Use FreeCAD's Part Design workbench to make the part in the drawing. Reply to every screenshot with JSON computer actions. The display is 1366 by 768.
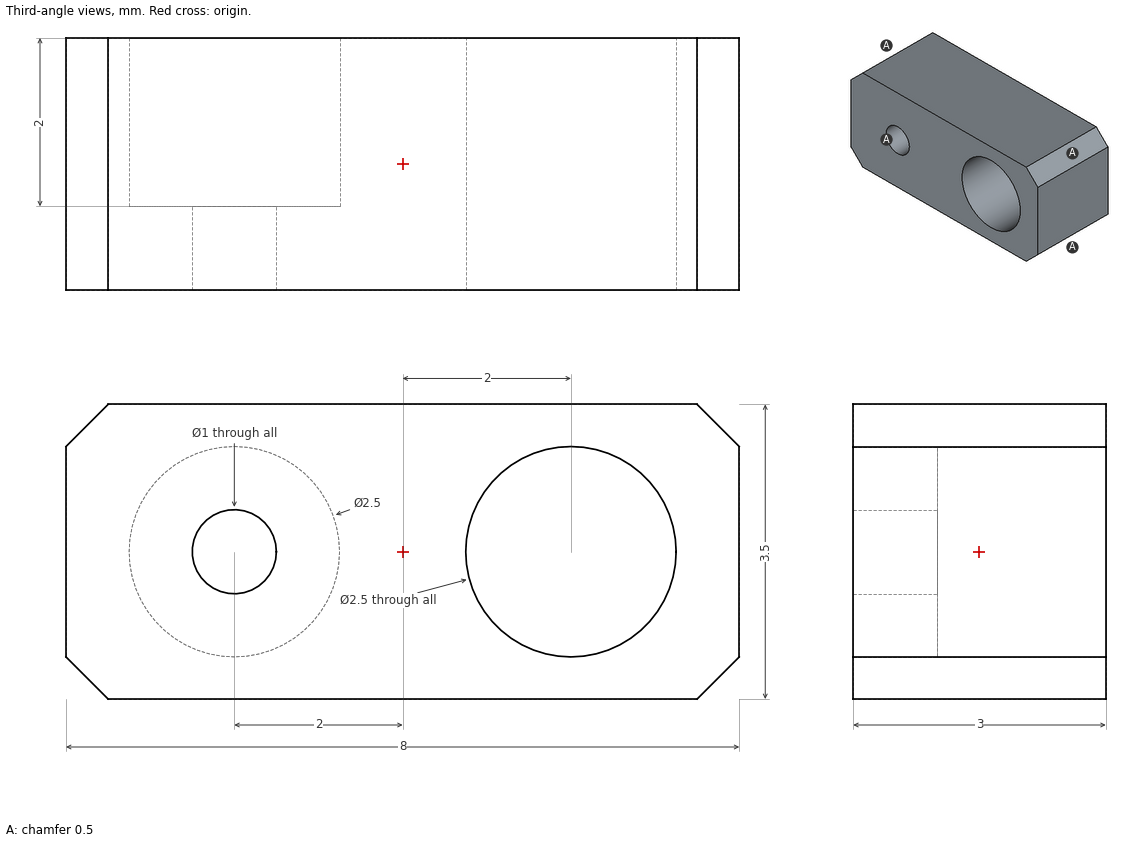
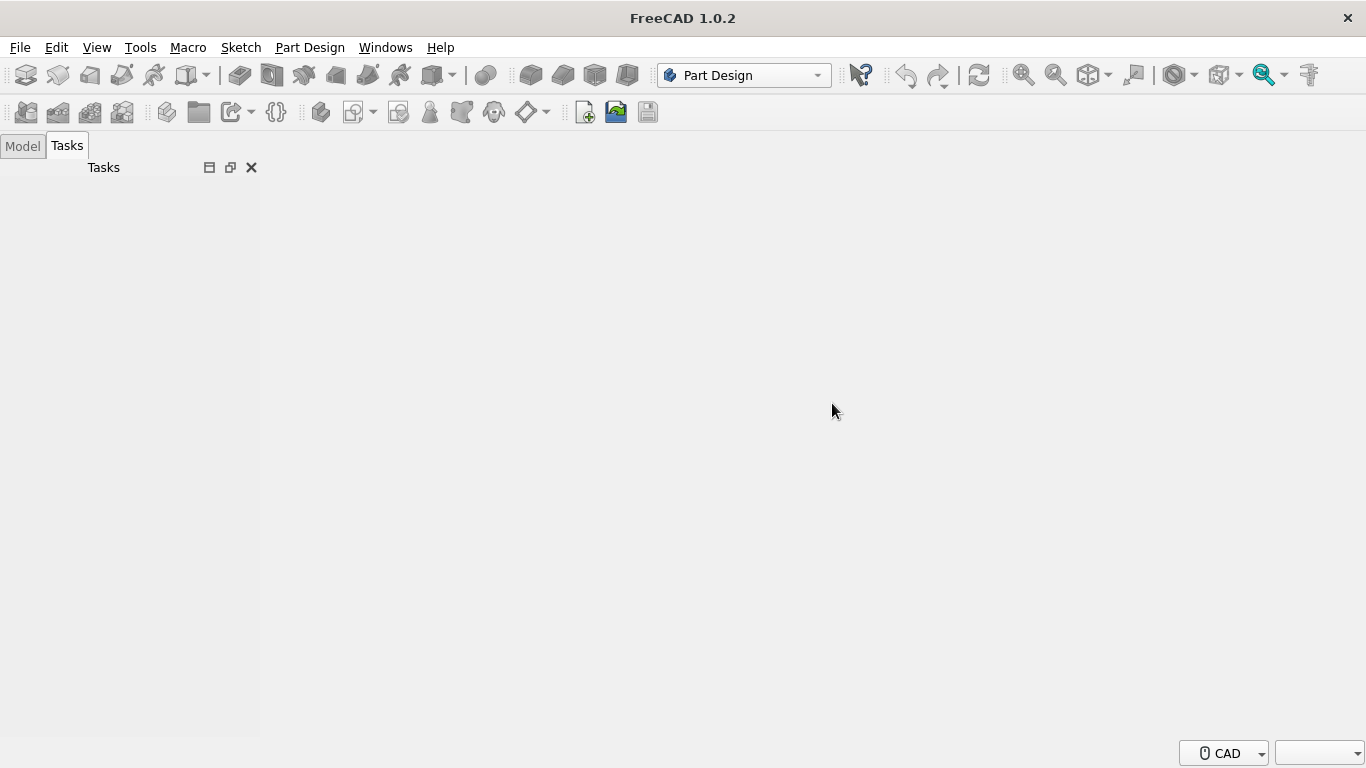
{"action": "left_click", "coordinate": [584, 112]}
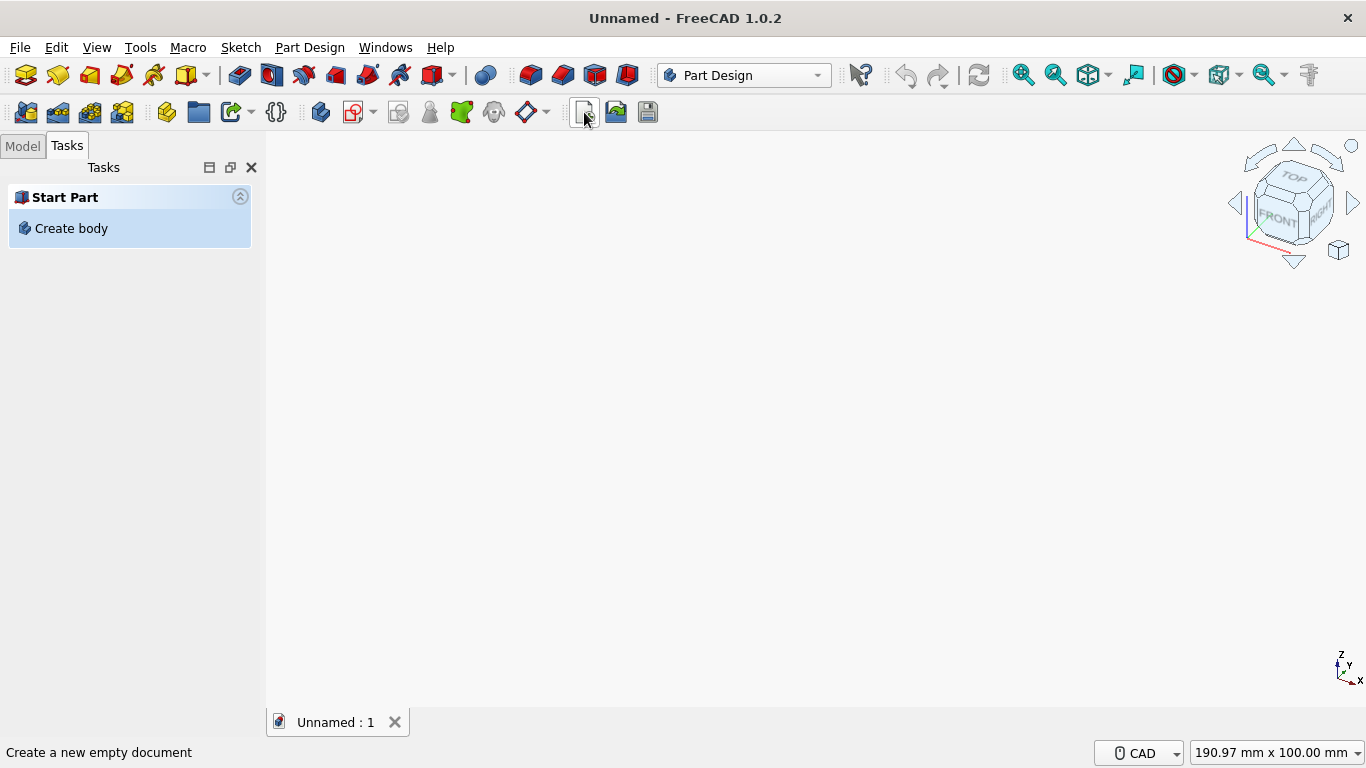
{"action": "left_click", "coordinate": [354, 112]}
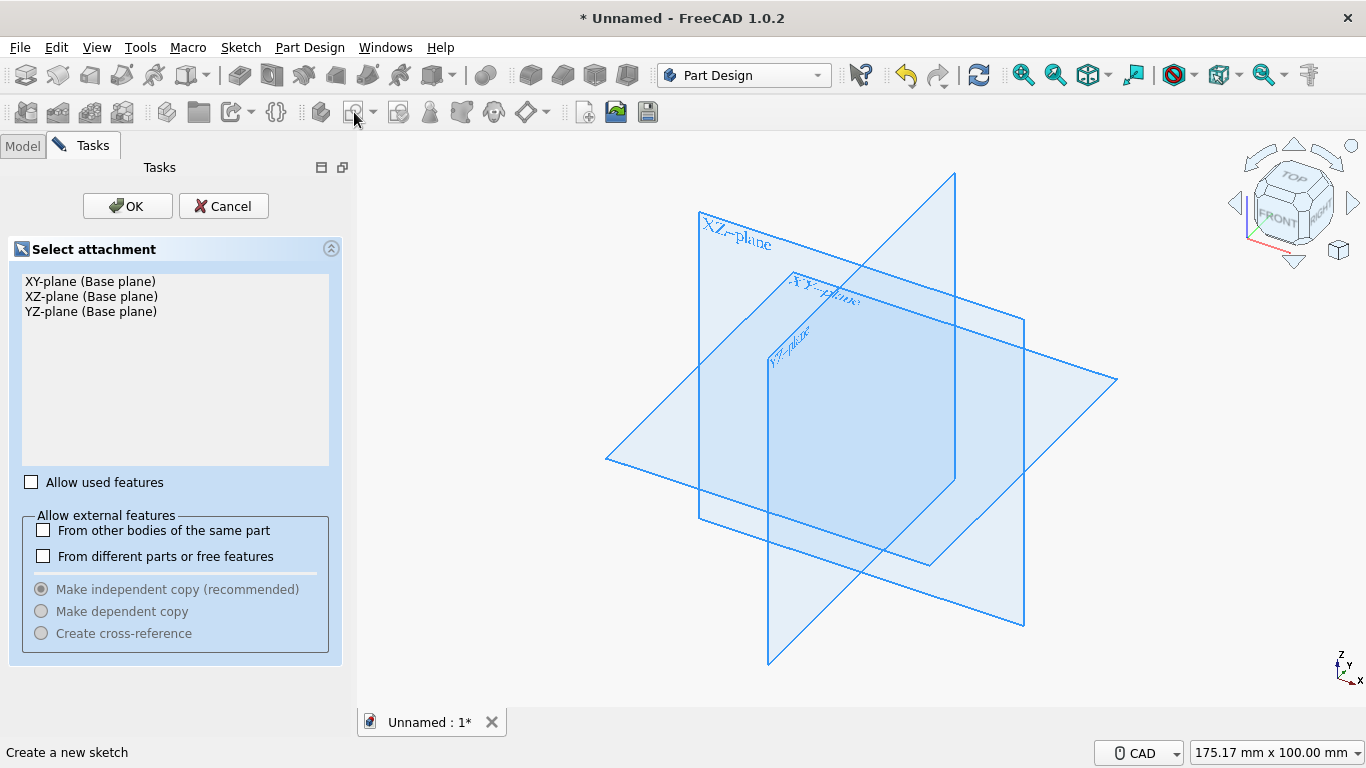
{"action": "left_click", "coordinate": [82, 296]}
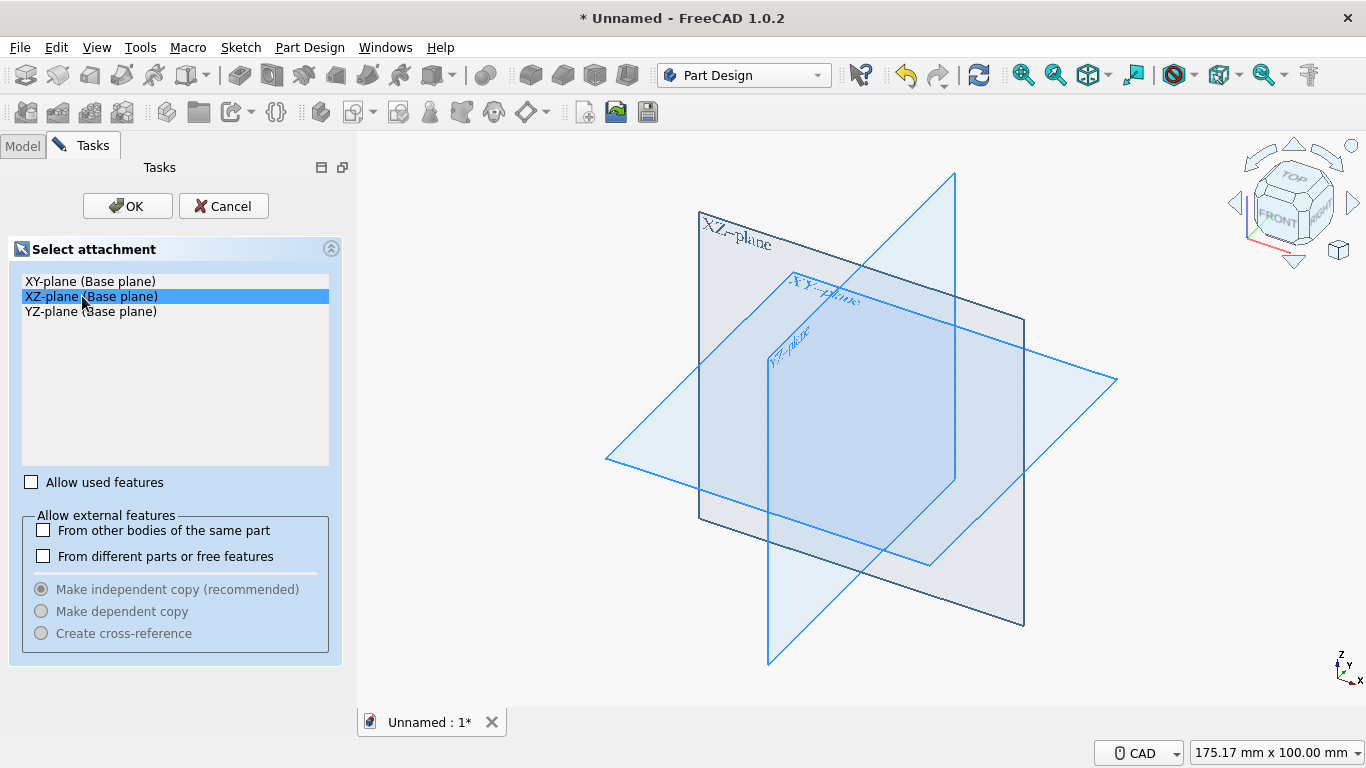
{"action": "left_click", "coordinate": [128, 206]}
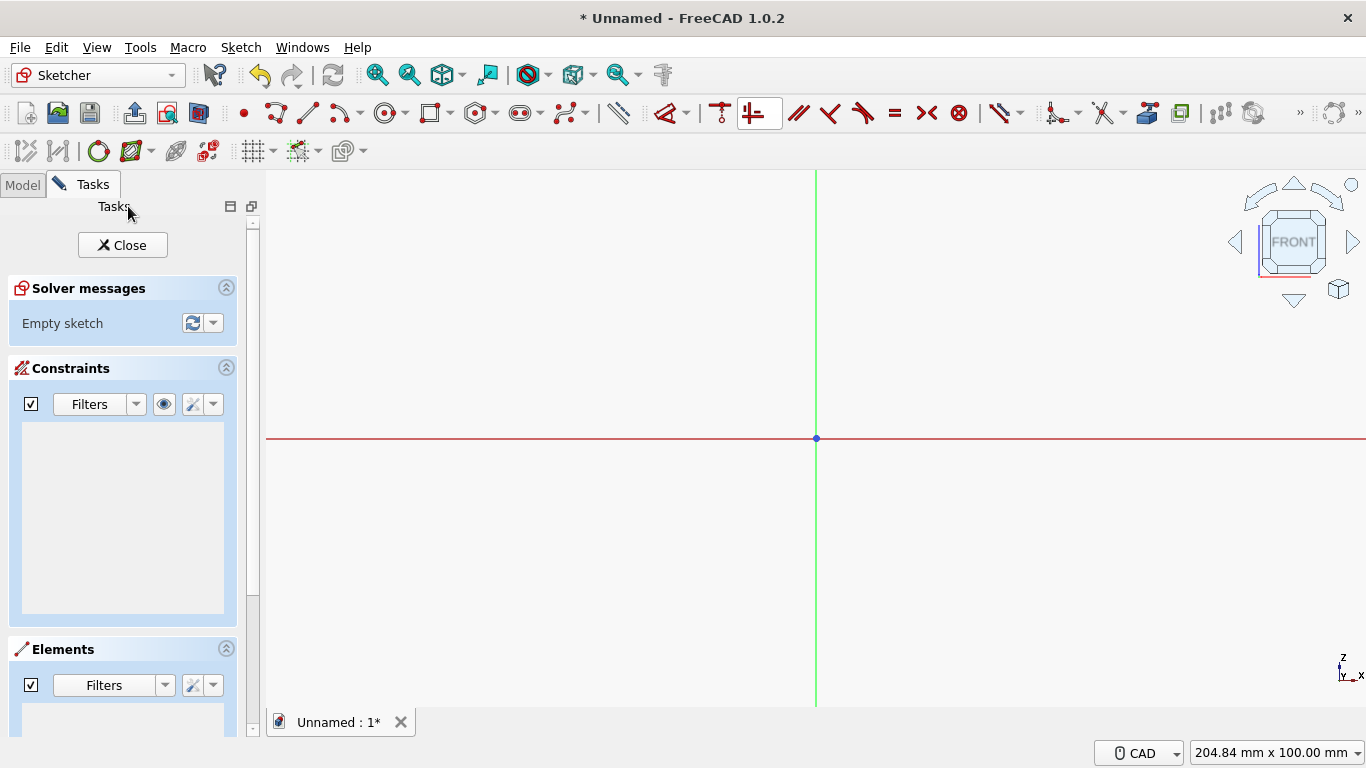
{"action": "scroll", "coordinate": [820, 438], "scroll_direction": "up", "scroll_amount": 14}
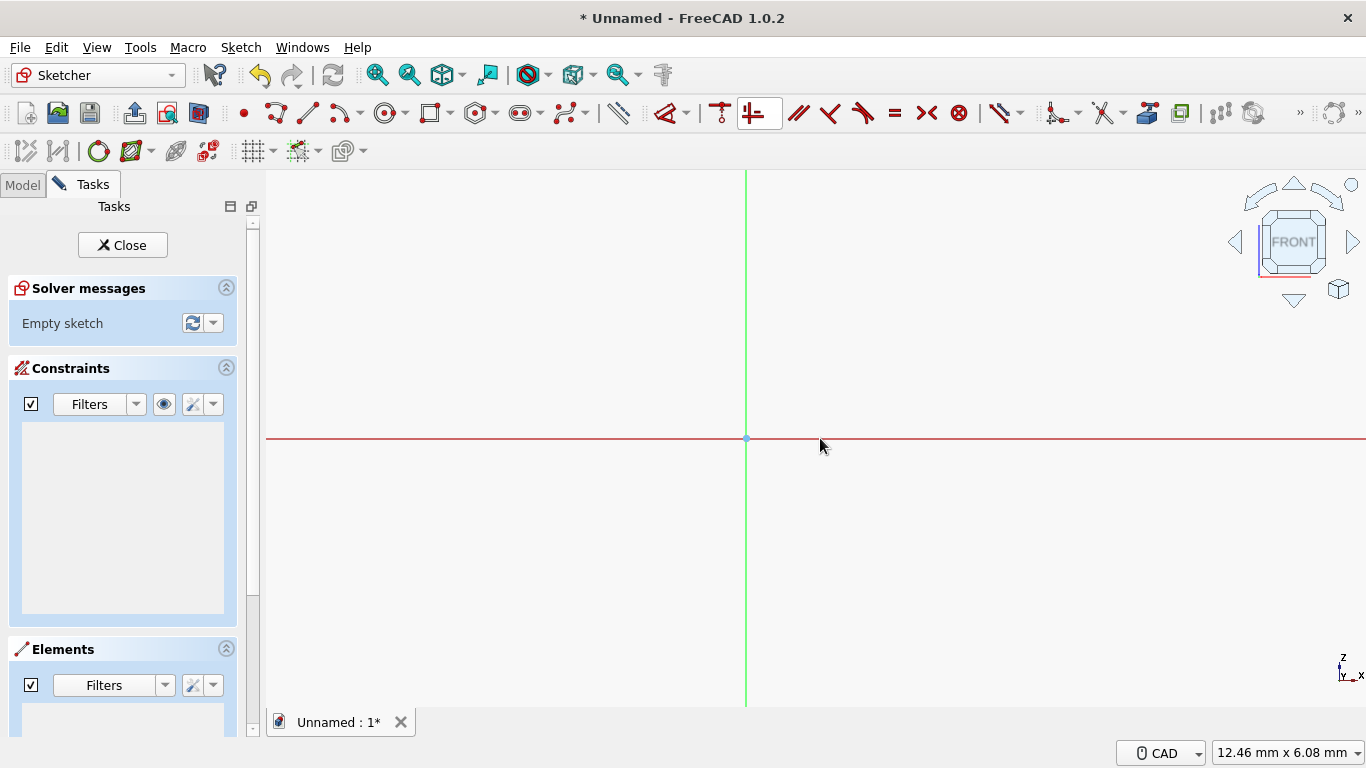
{"action": "key", "text": "g v"}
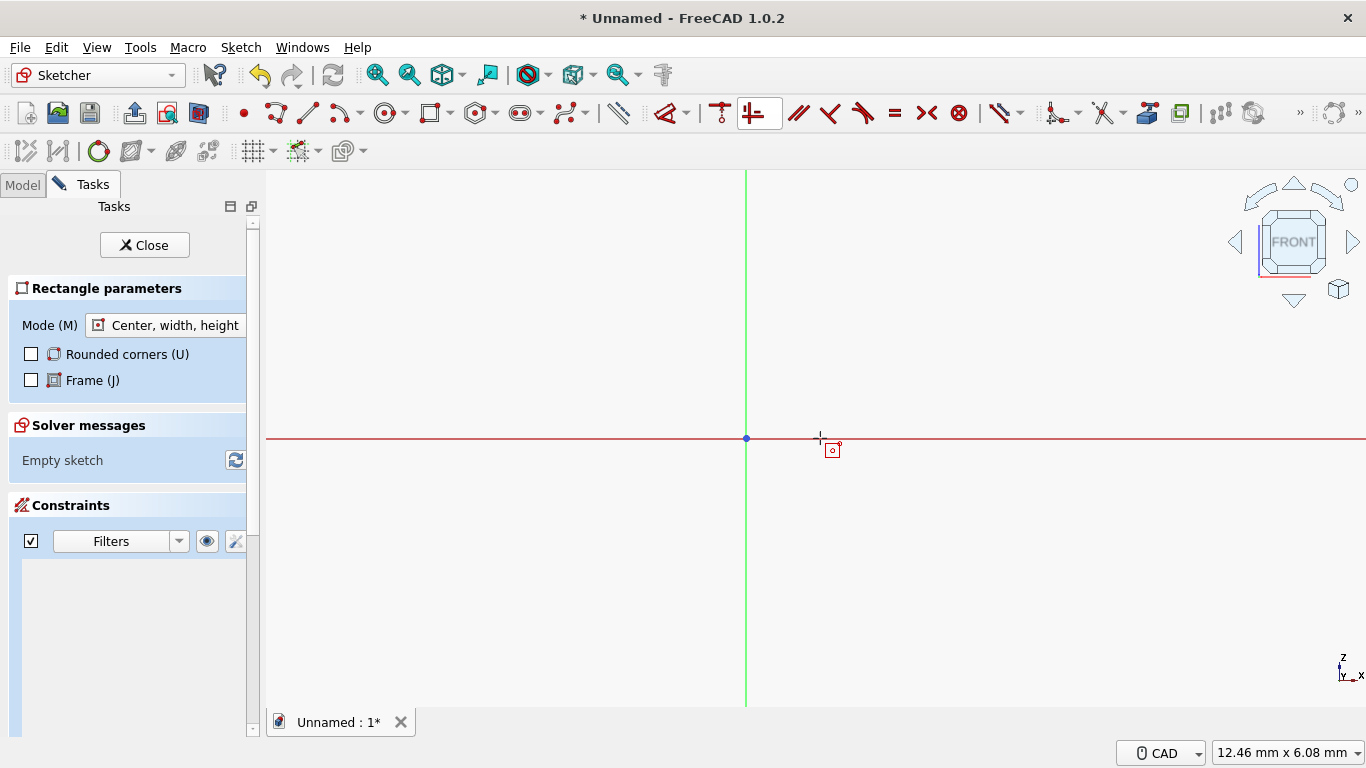
{"action": "left_click", "coordinate": [746, 438]}
{"action": "left_click", "coordinate": [1100, 284]}
{"action": "key", "text": "Escape"}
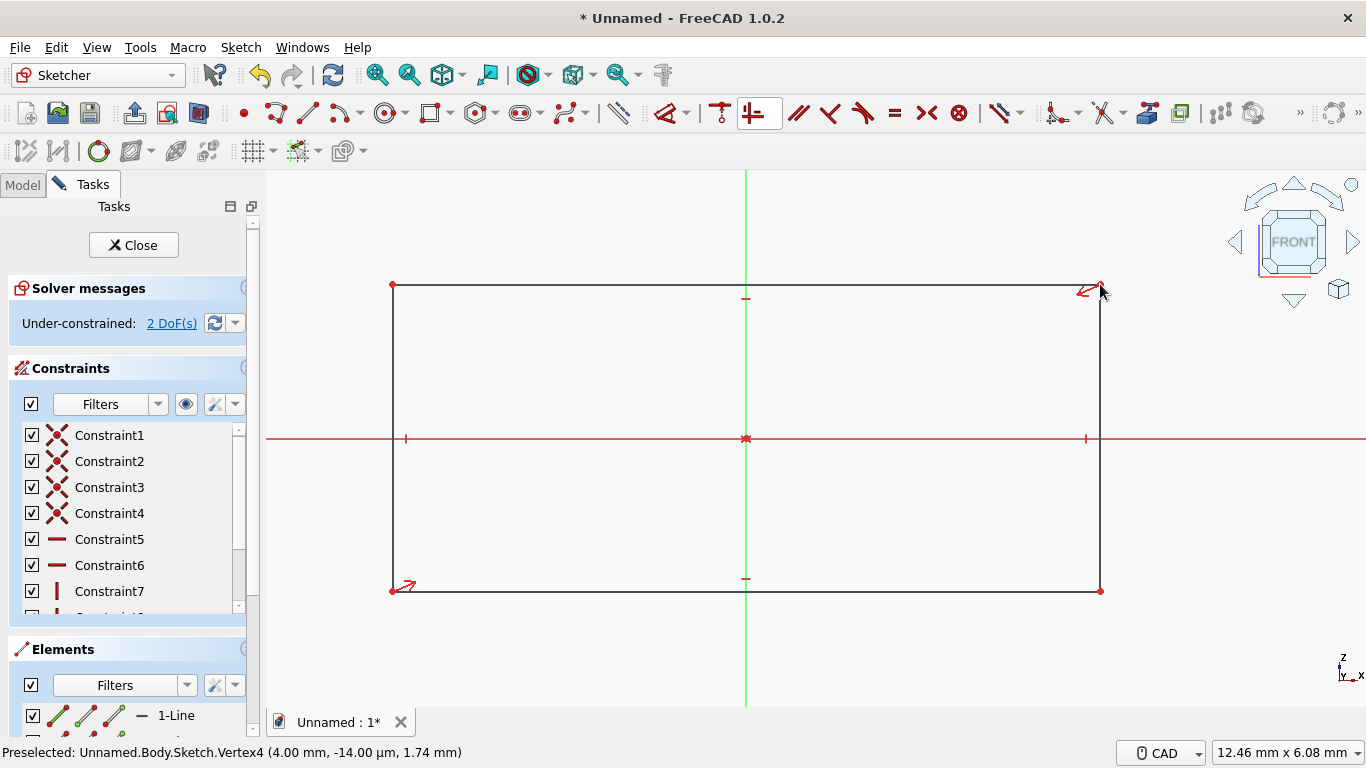
{"action": "left_click", "coordinate": [666, 114]}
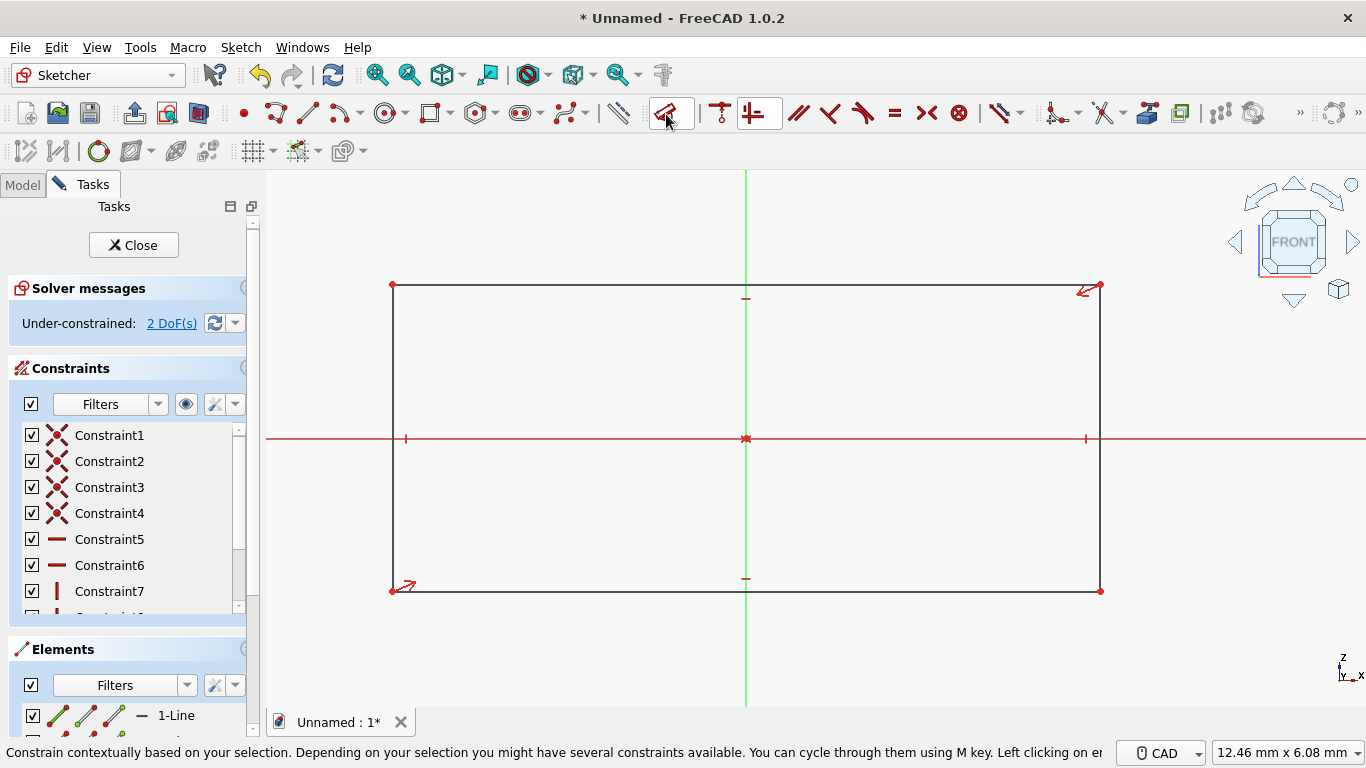
{"action": "left_click", "coordinate": [605, 592]}
{"action": "left_click", "coordinate": [584, 626]}